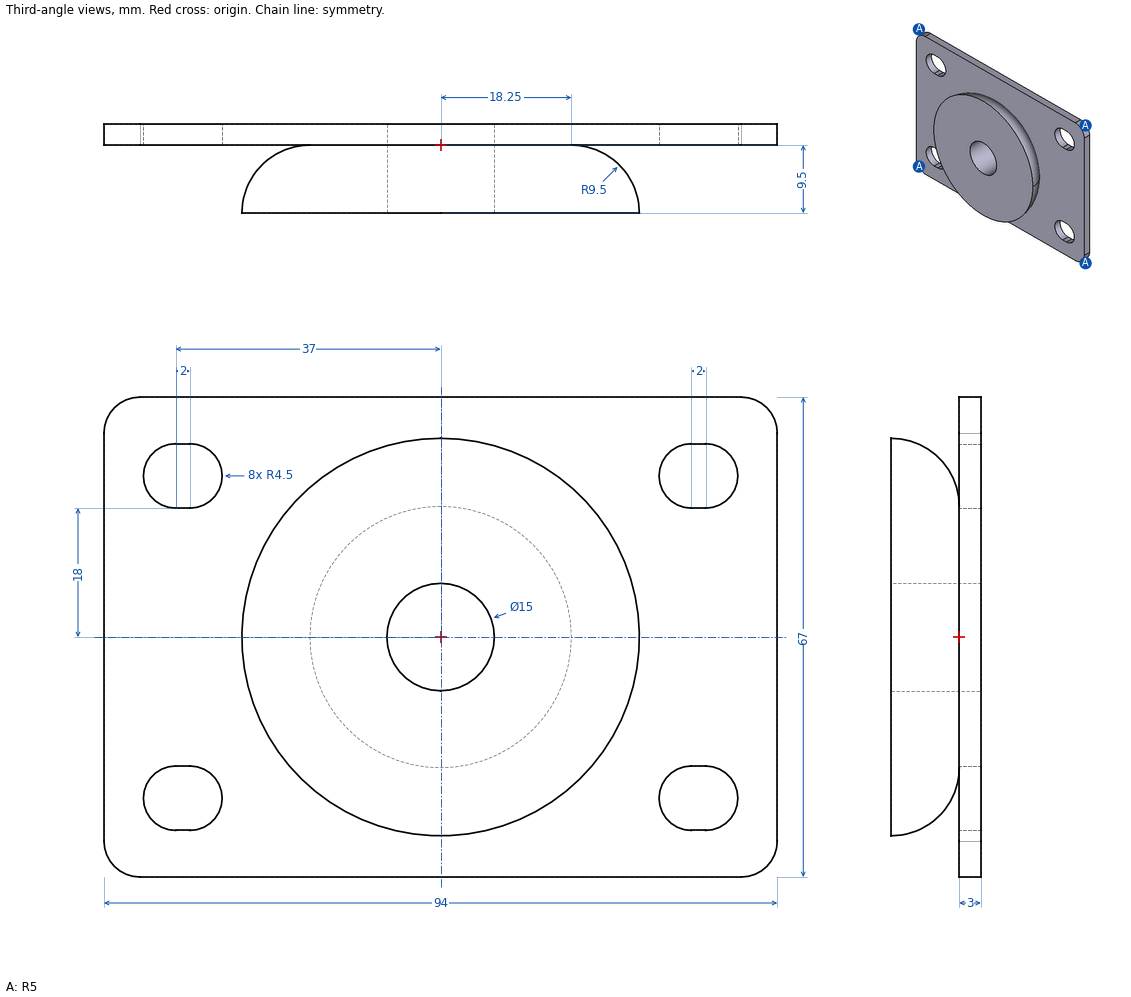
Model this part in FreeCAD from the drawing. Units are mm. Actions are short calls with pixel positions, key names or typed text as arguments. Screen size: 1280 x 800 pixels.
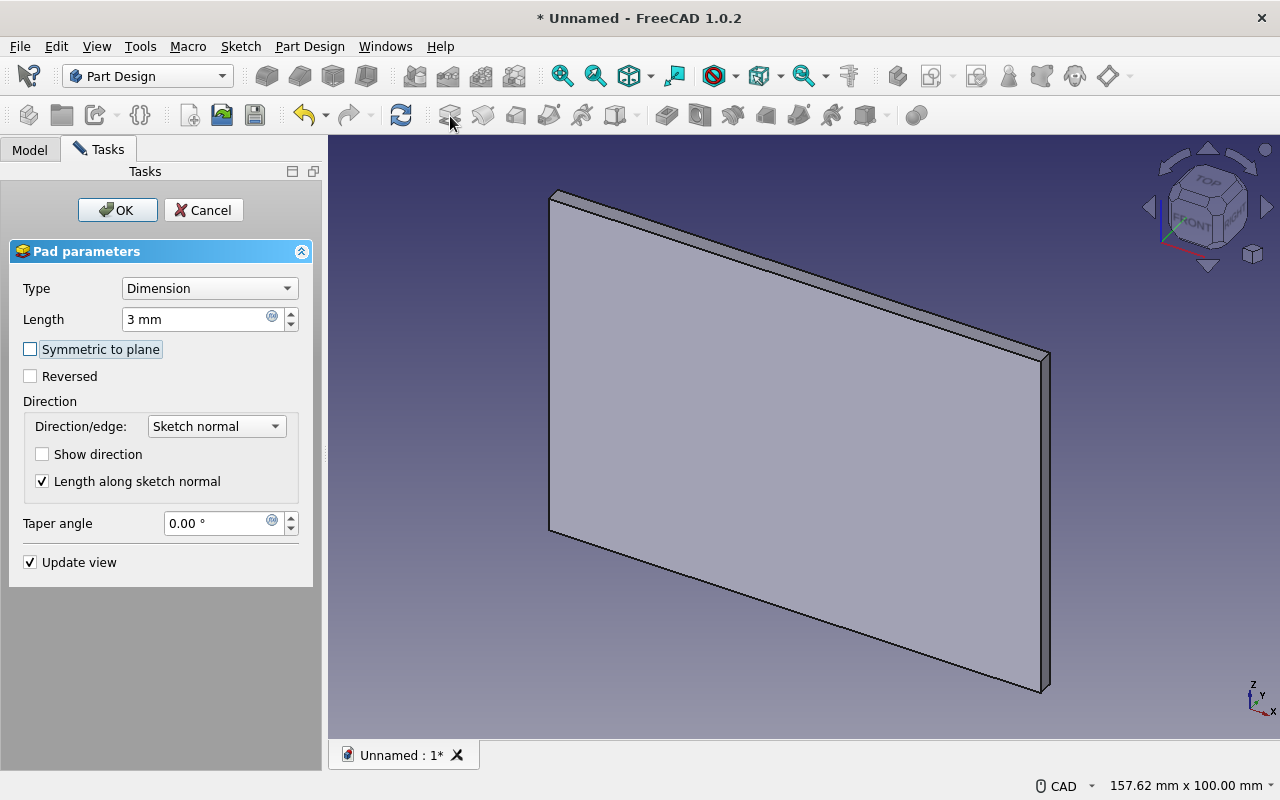
click(31, 376)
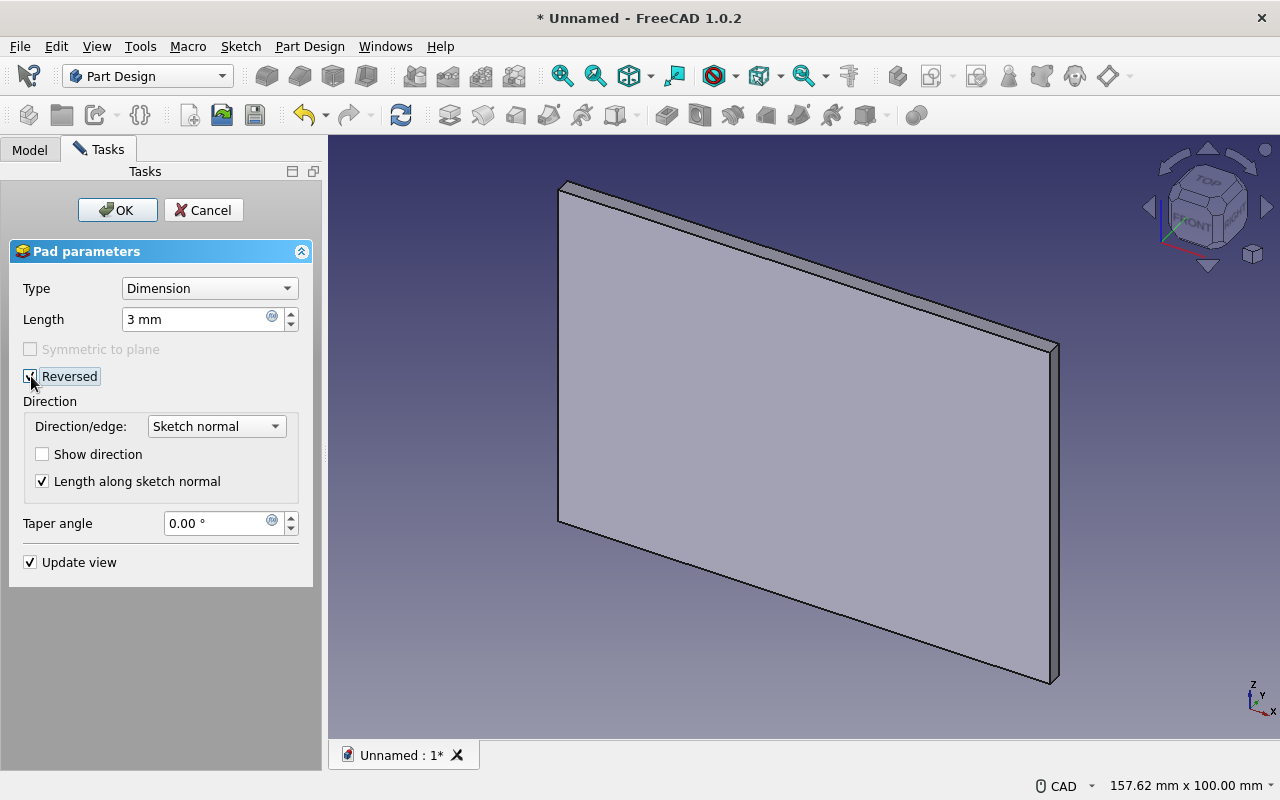
click(118, 210)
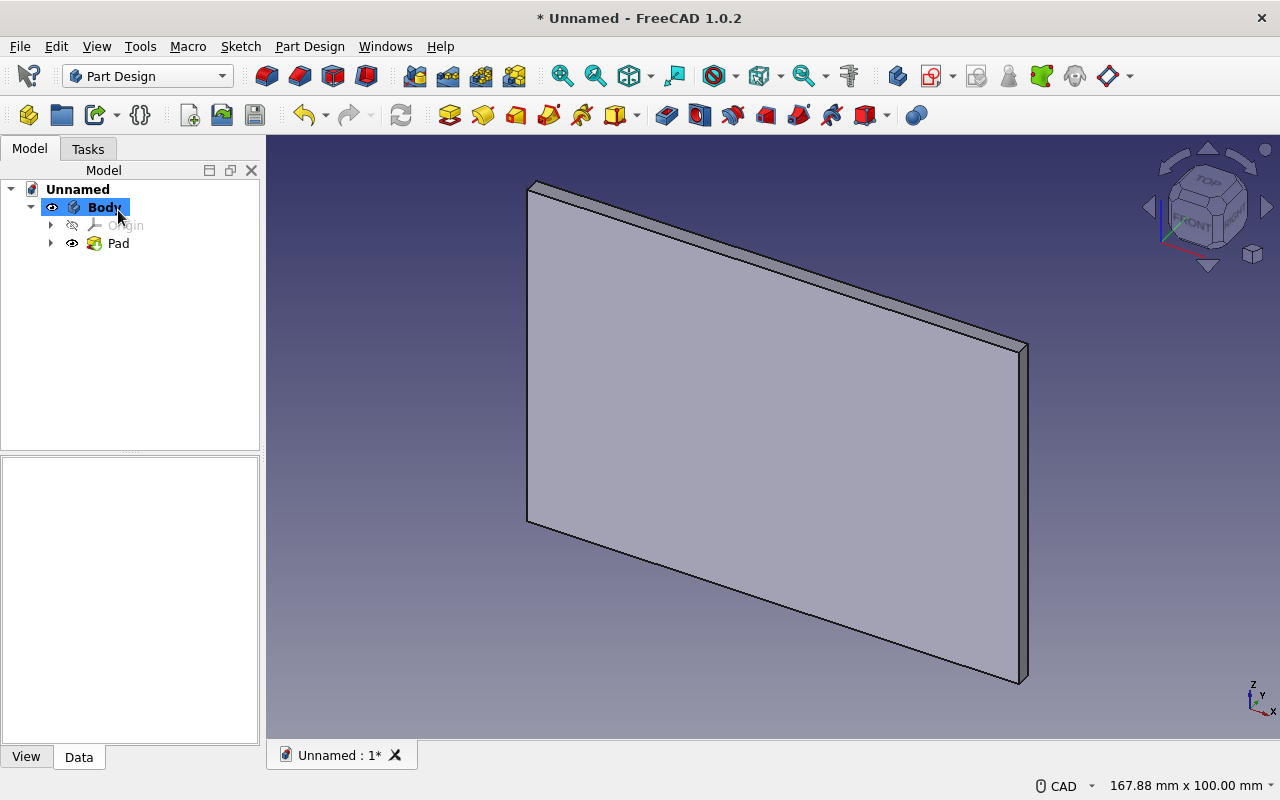
click(1024, 346)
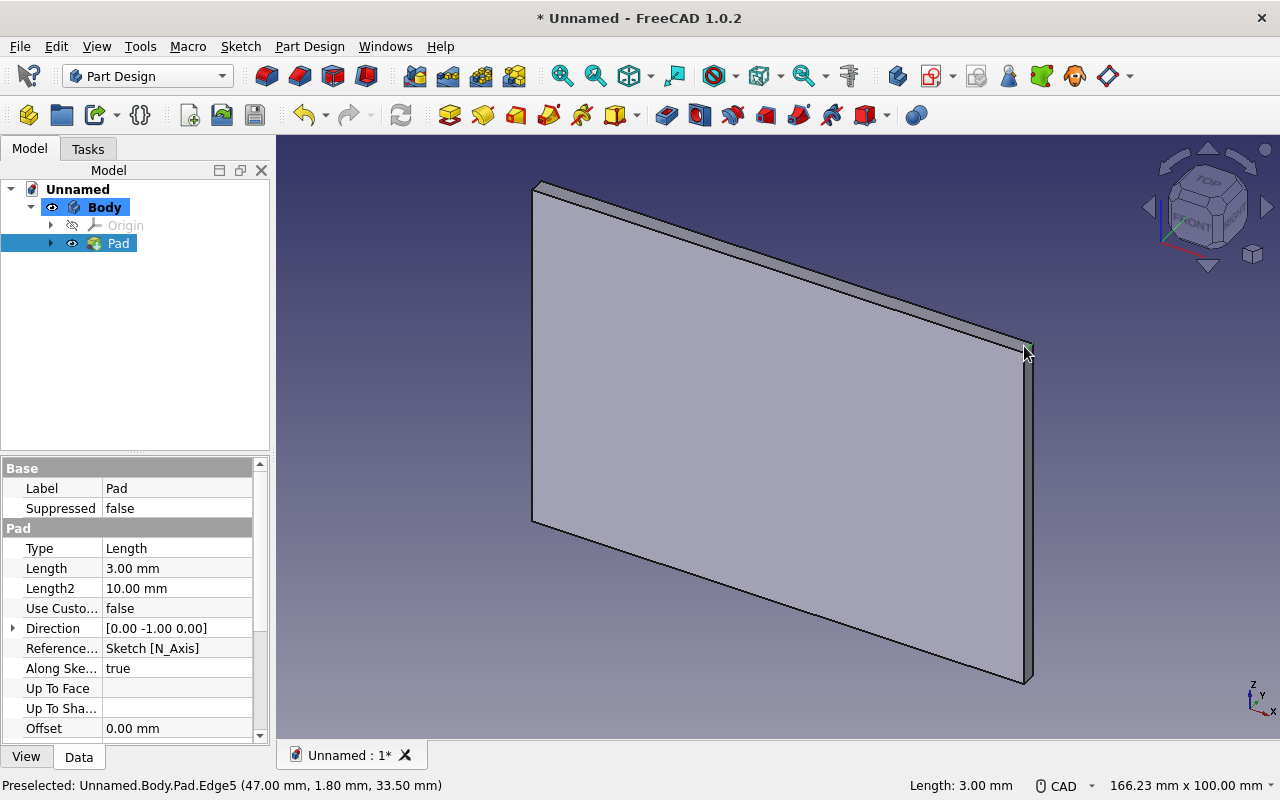
scroll(537, 516, up, 4)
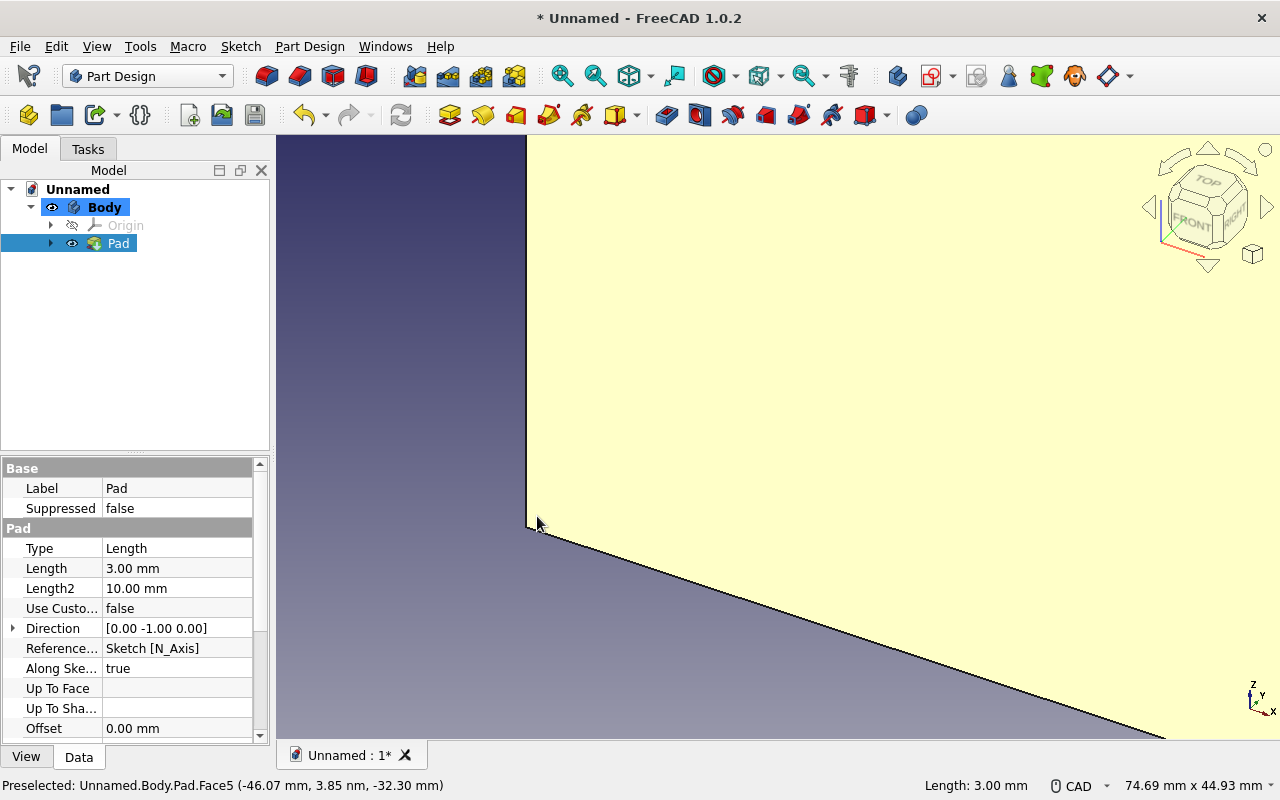
key(v)
key(f)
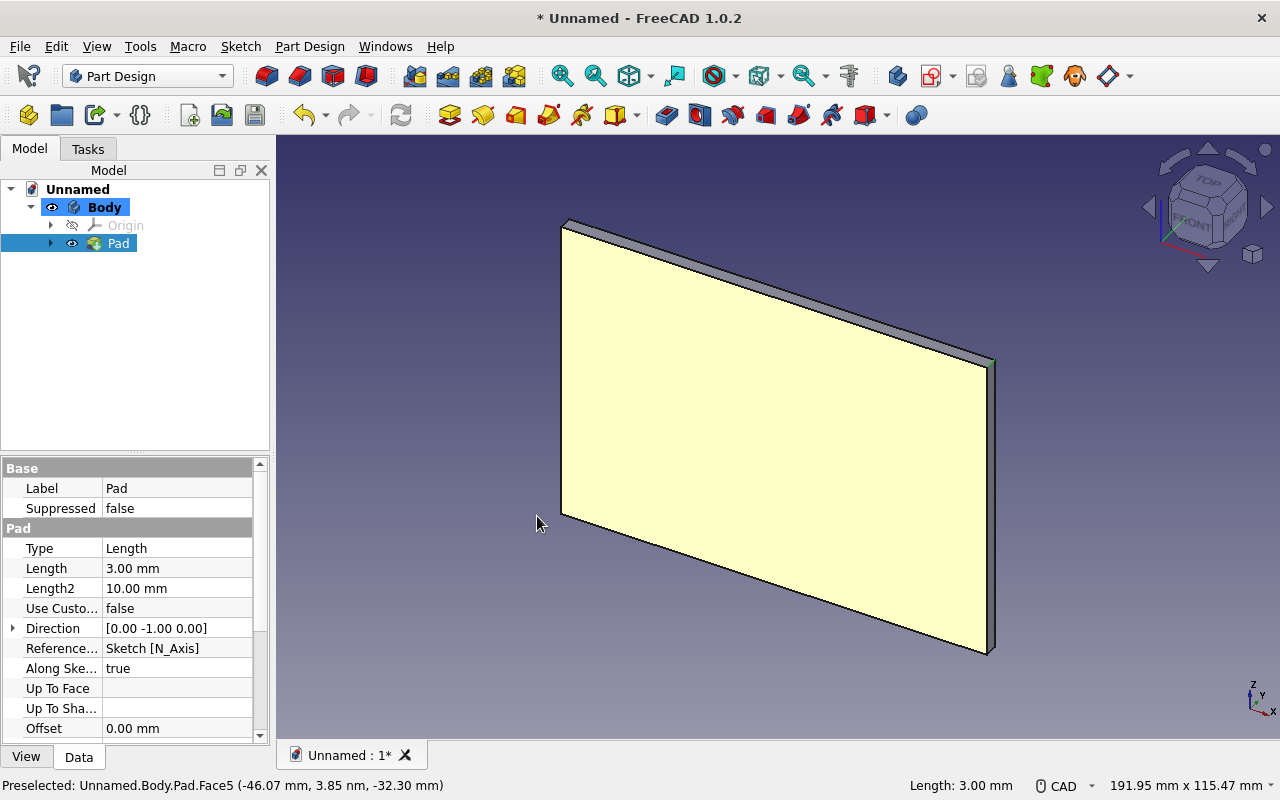
key(0)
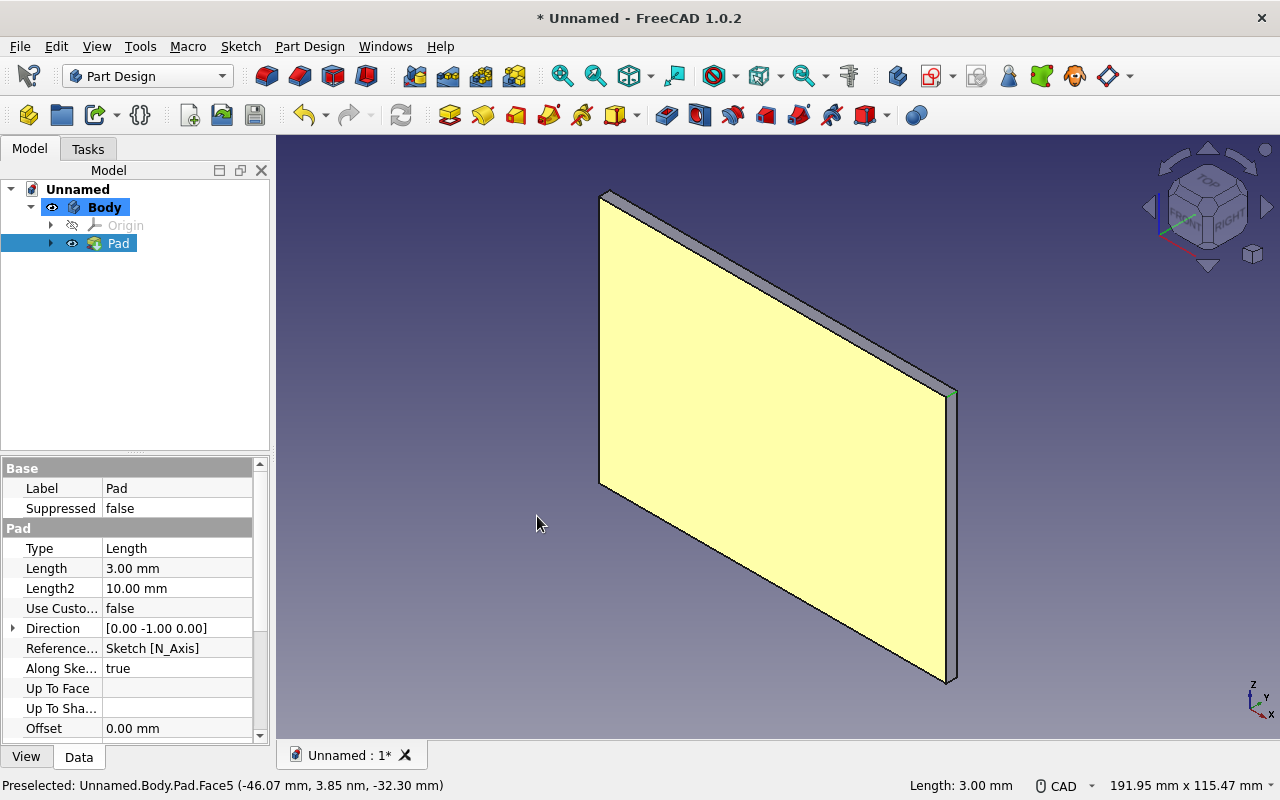
scroll(604, 479, up, 5)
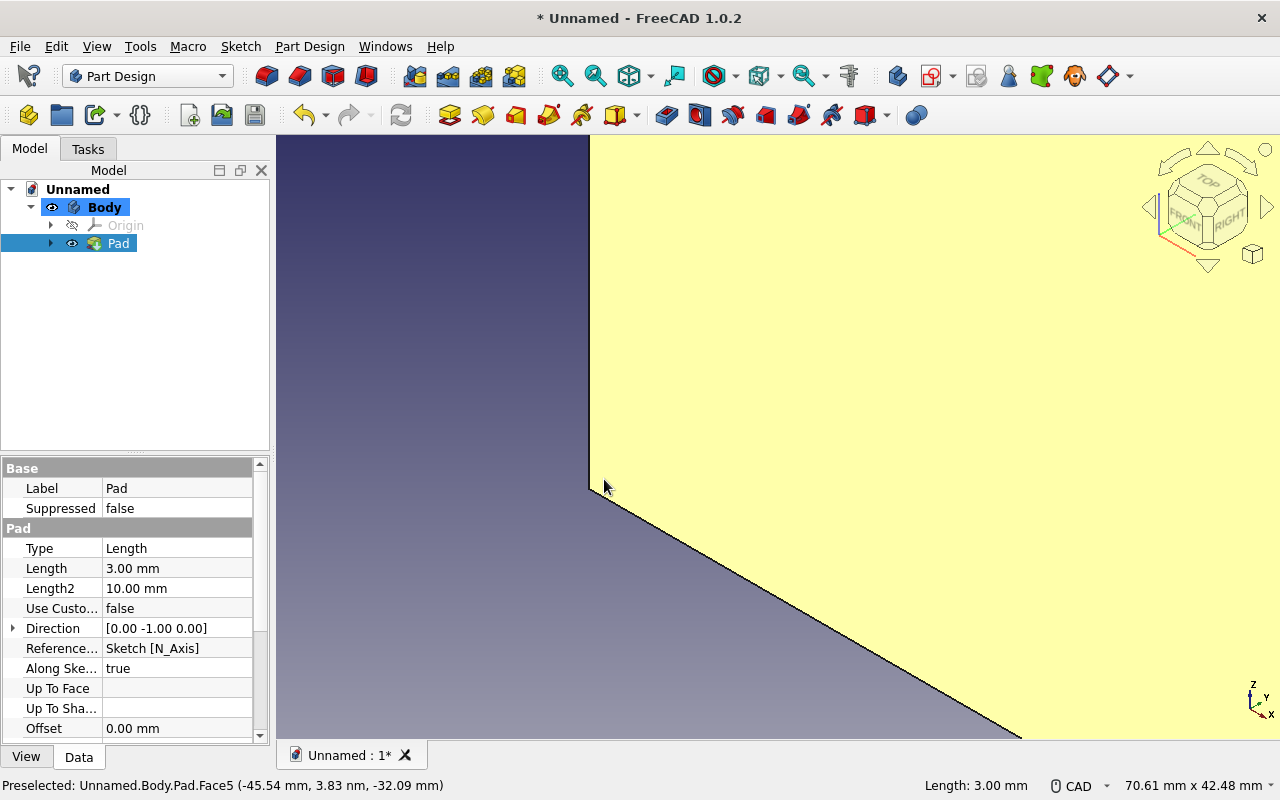
key(v)
key(f)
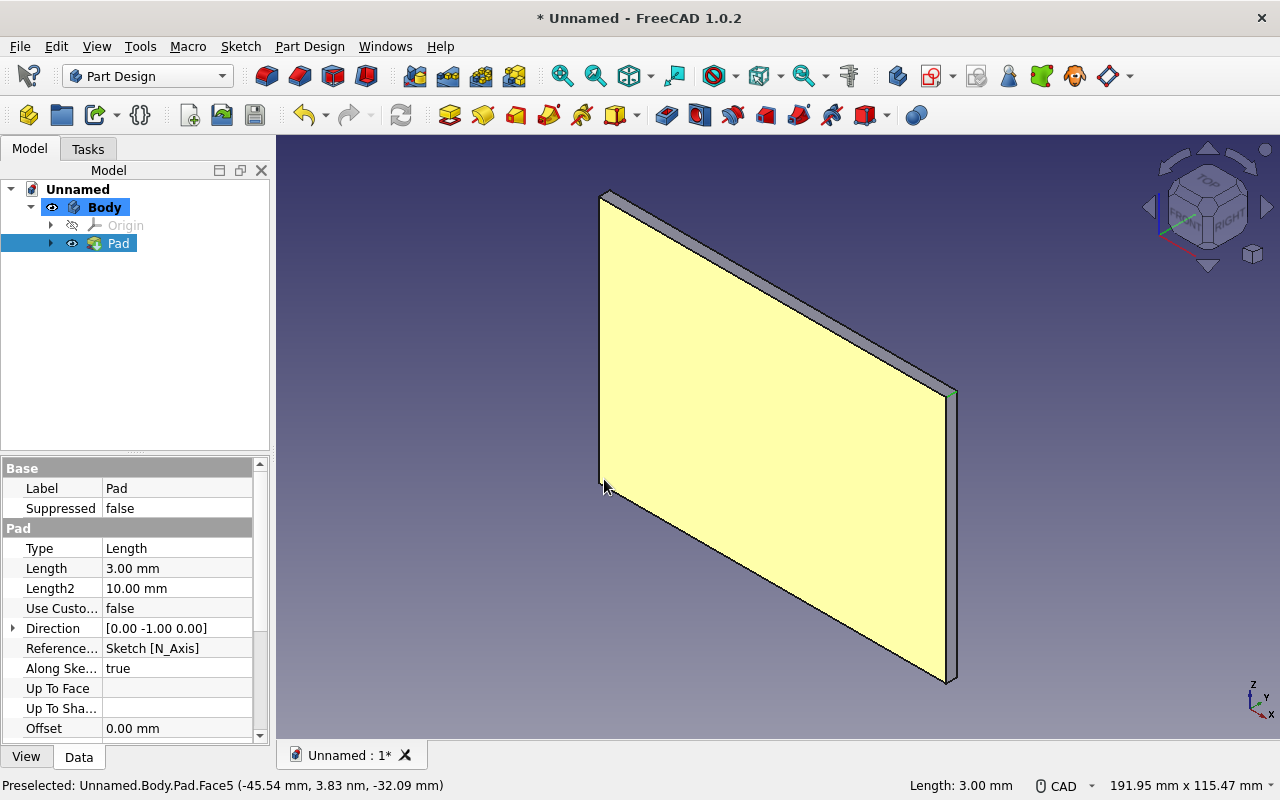
key(2)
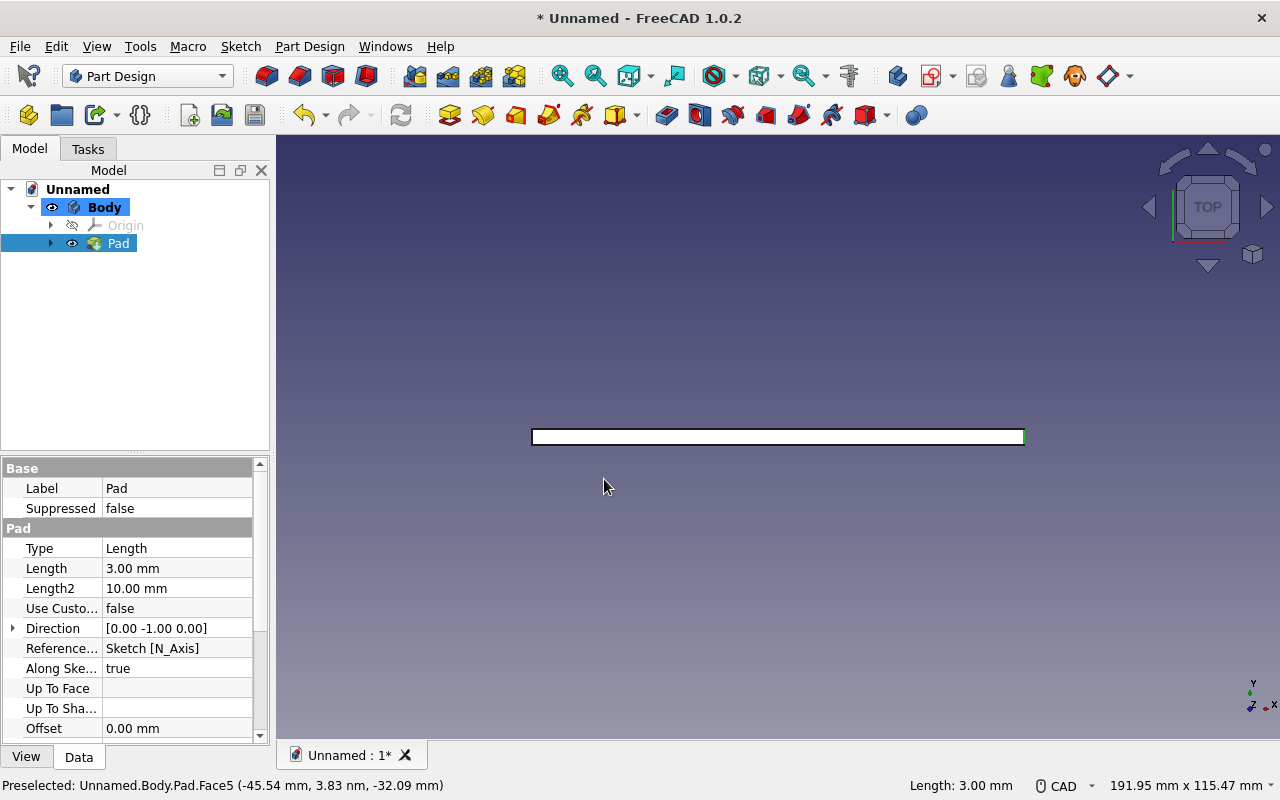
click(532, 436, ctrl)